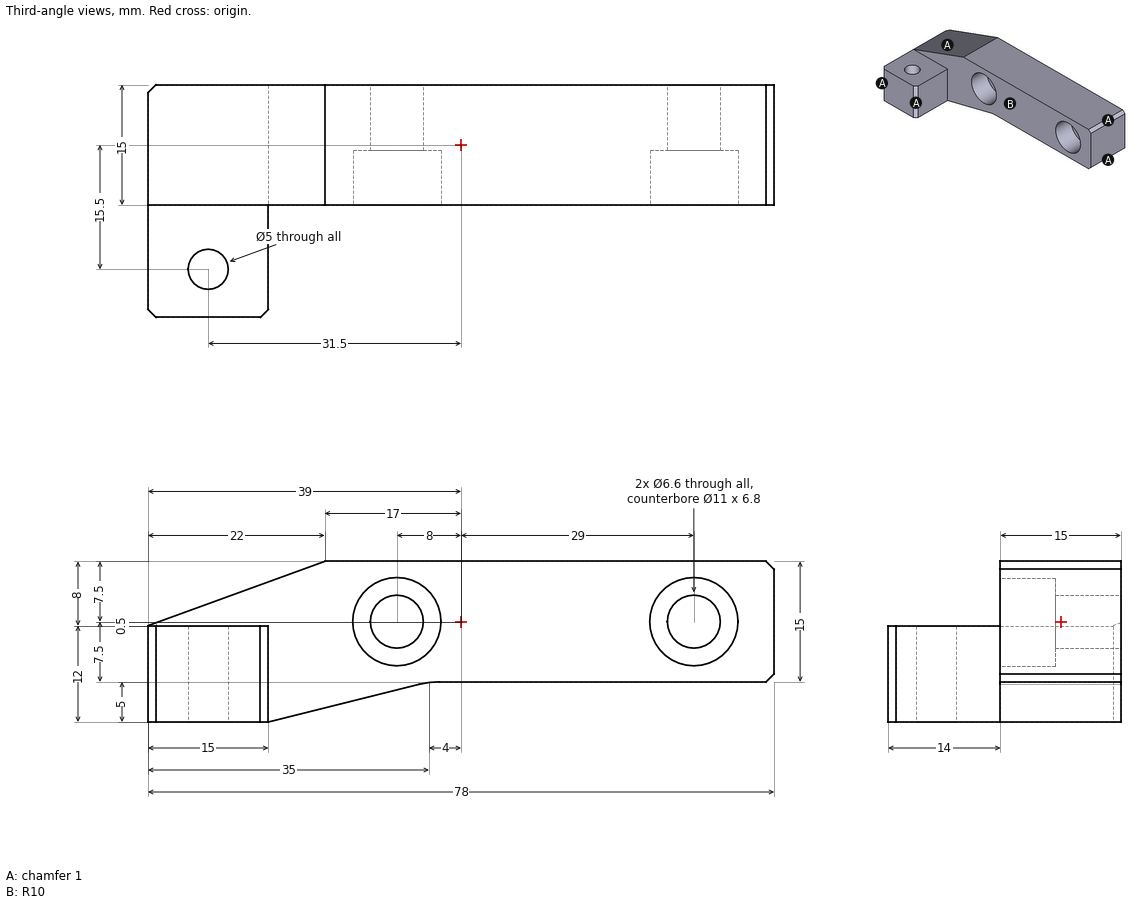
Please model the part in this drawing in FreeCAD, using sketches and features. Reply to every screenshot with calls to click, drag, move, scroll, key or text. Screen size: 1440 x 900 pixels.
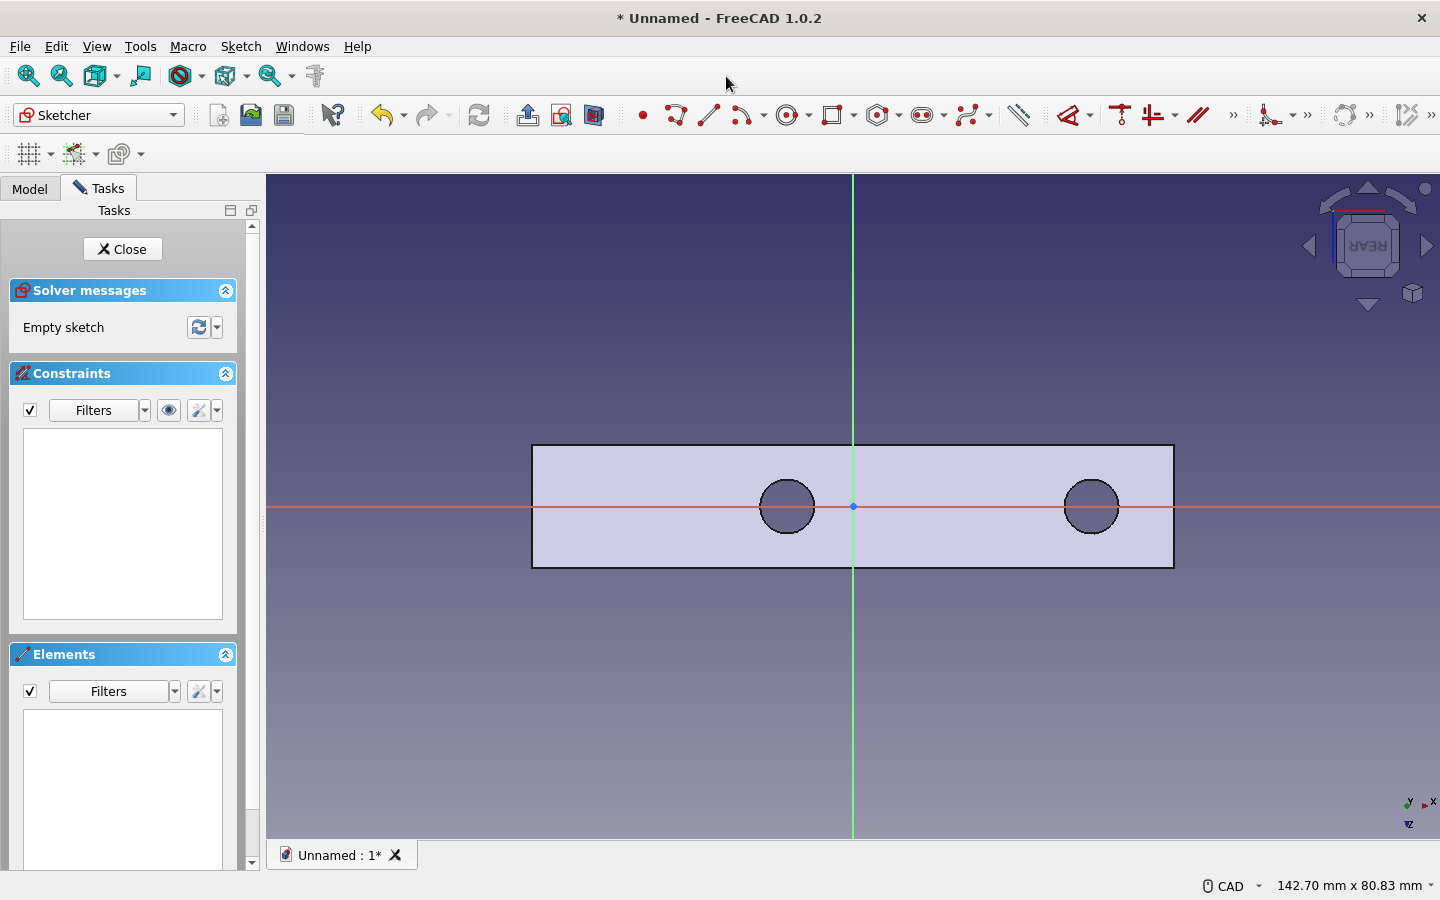
scroll(618, 413, up, 4)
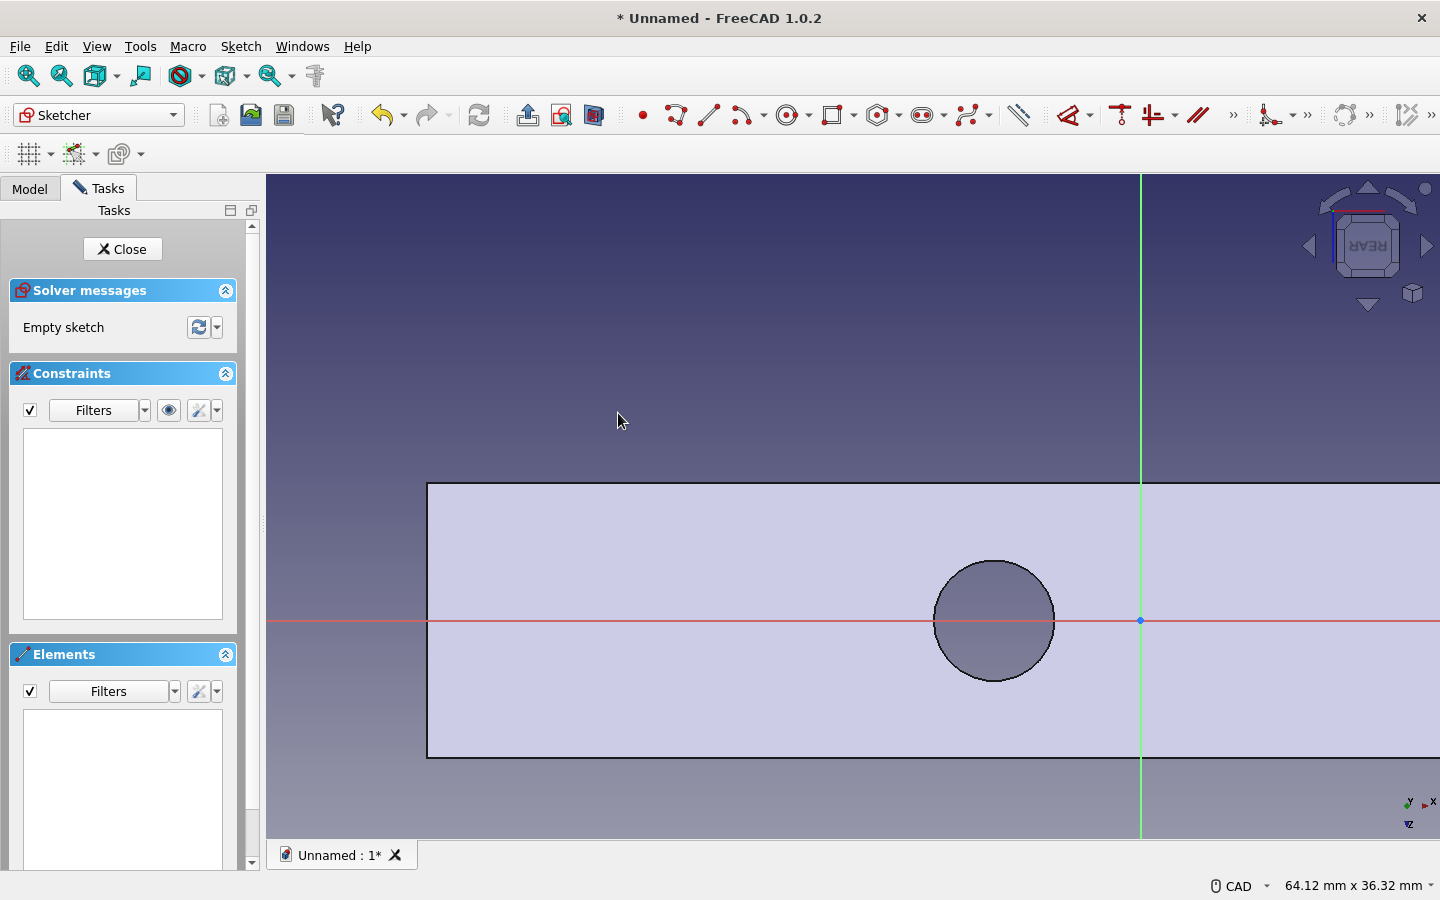
key(g)
key(m)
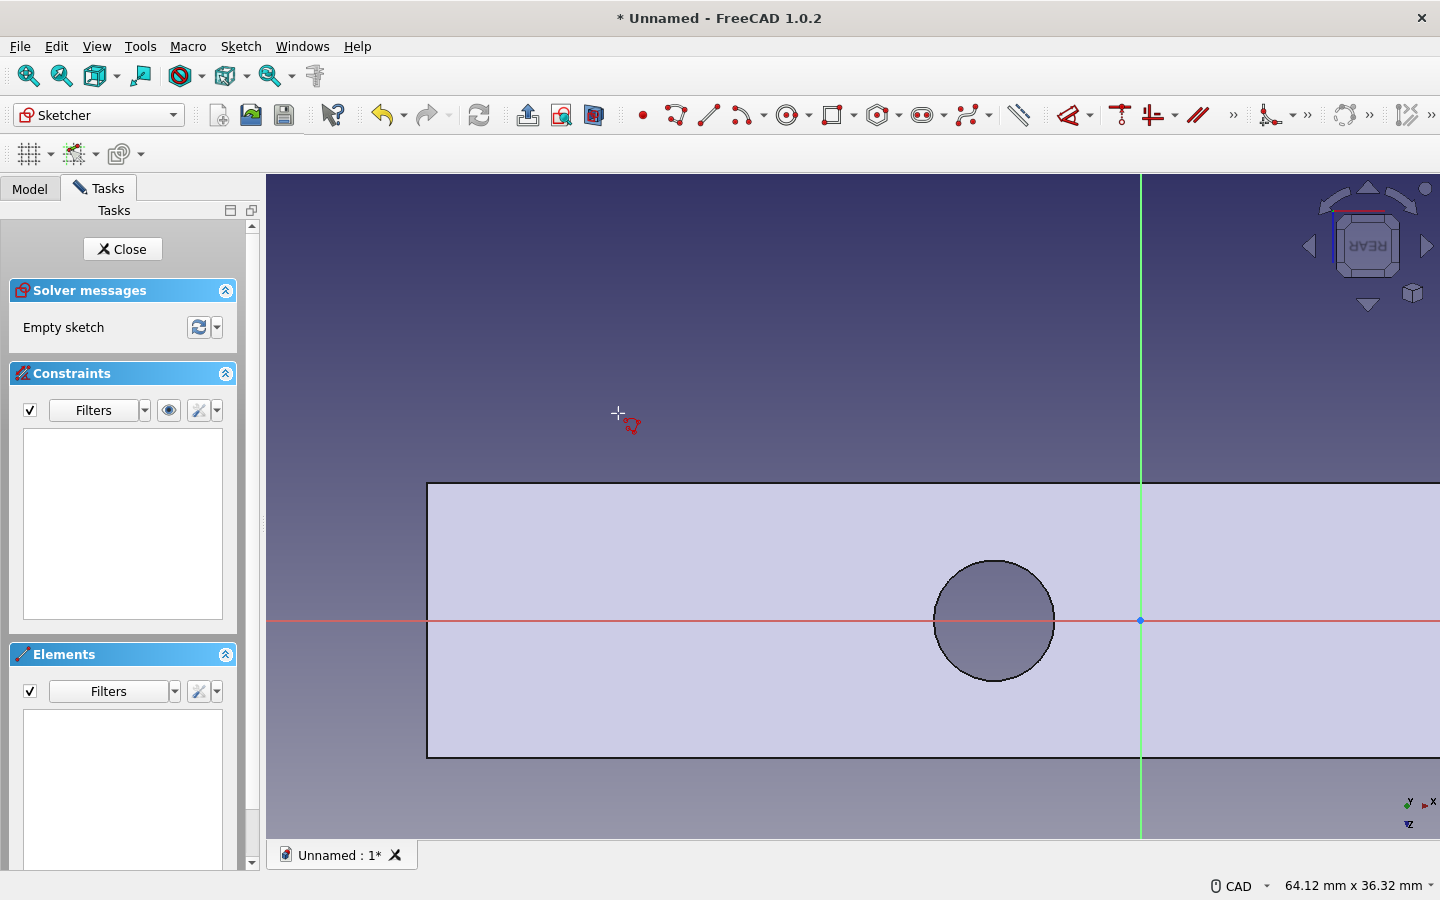
click(1067, 483)
click(701, 392)
click(427, 392)
click(427, 483)
click(1067, 484)
key(Escape)
key(Escape)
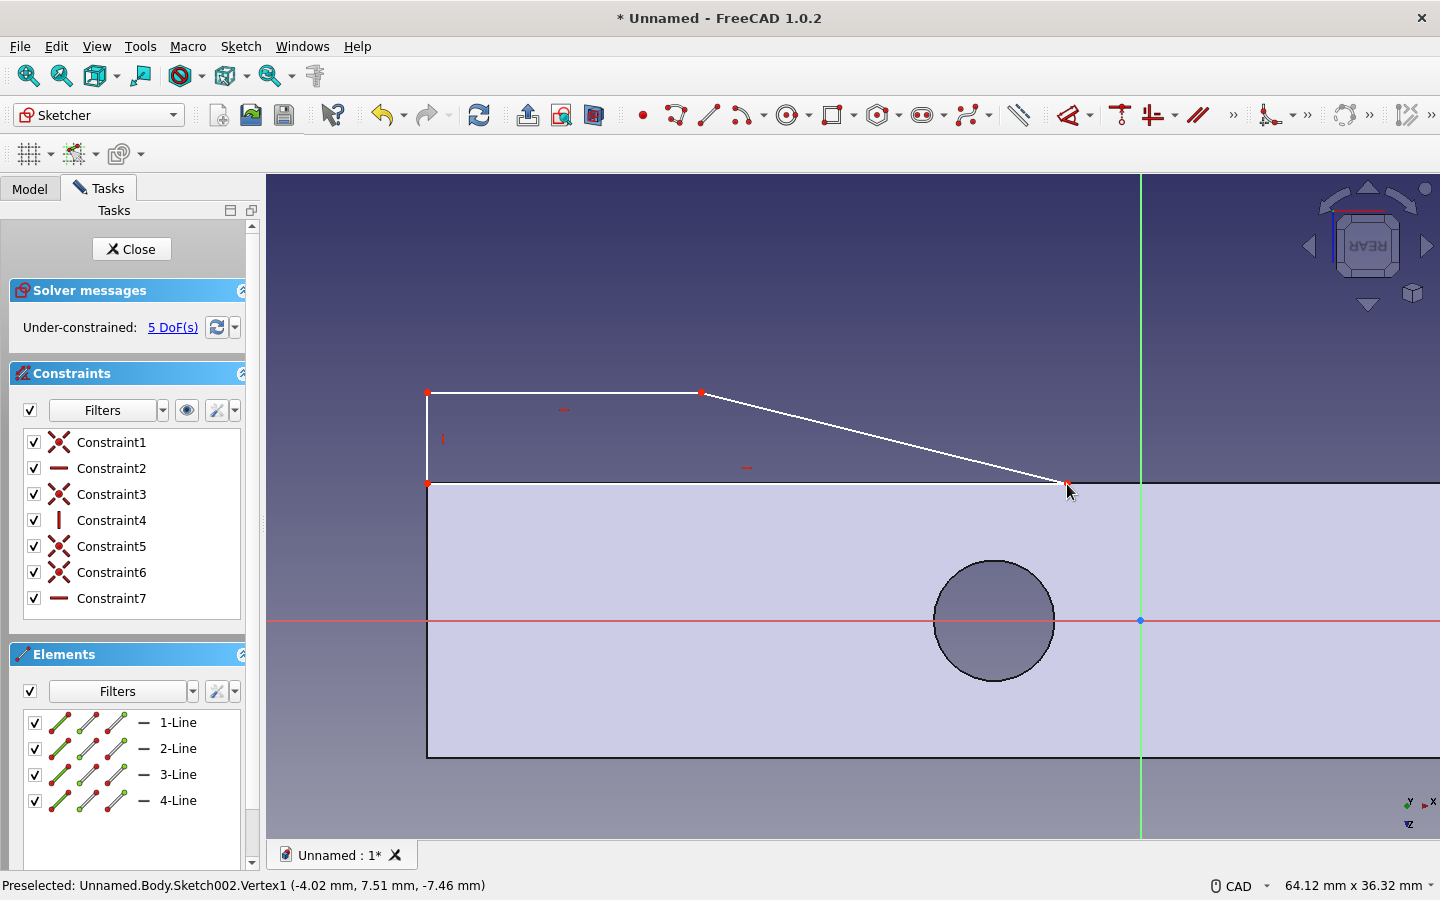
click(427, 420)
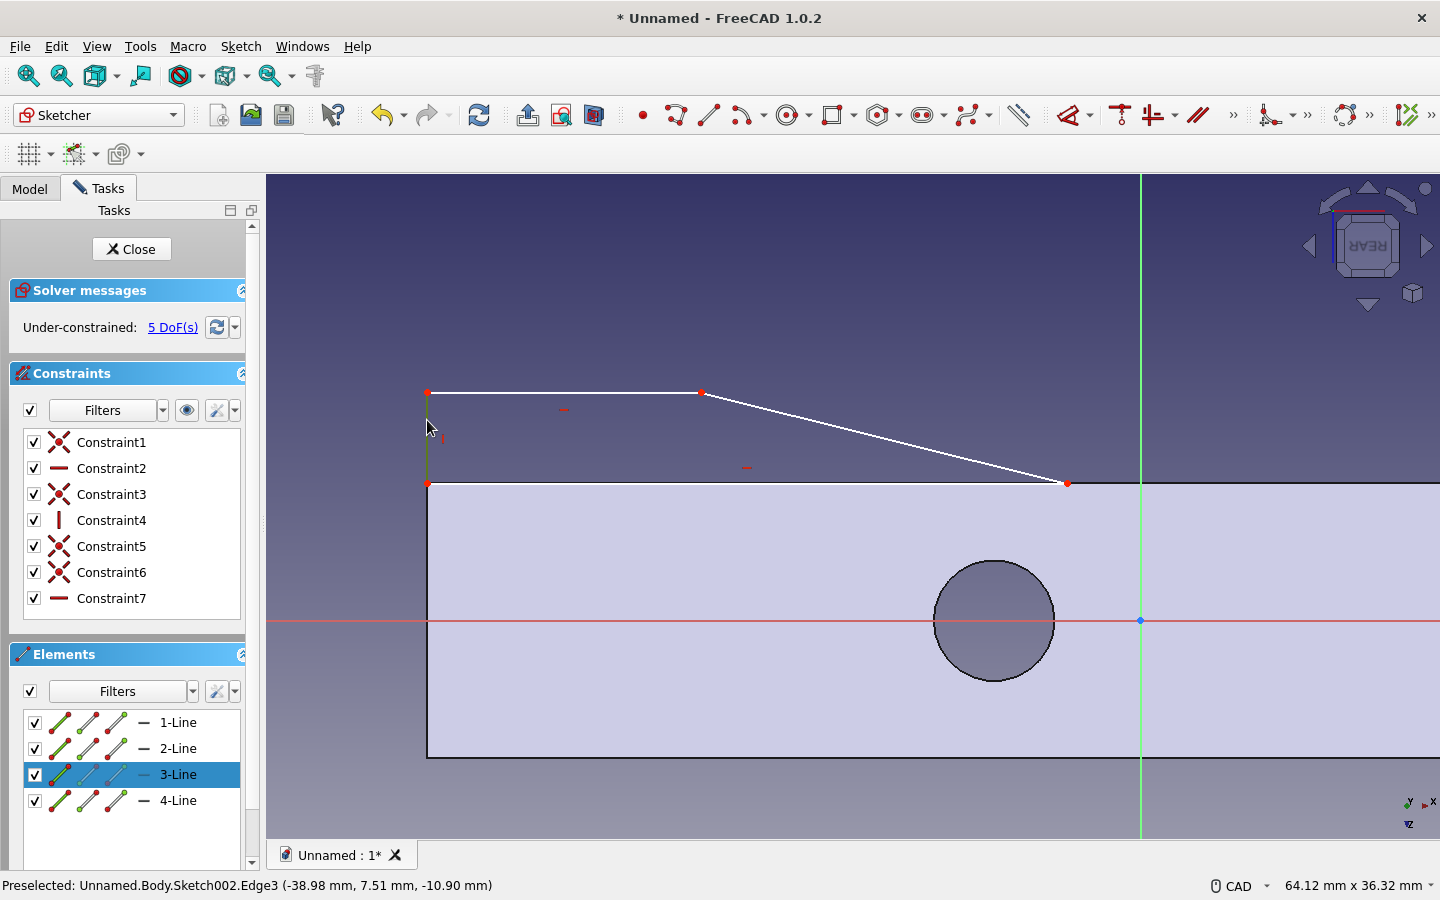
key(i)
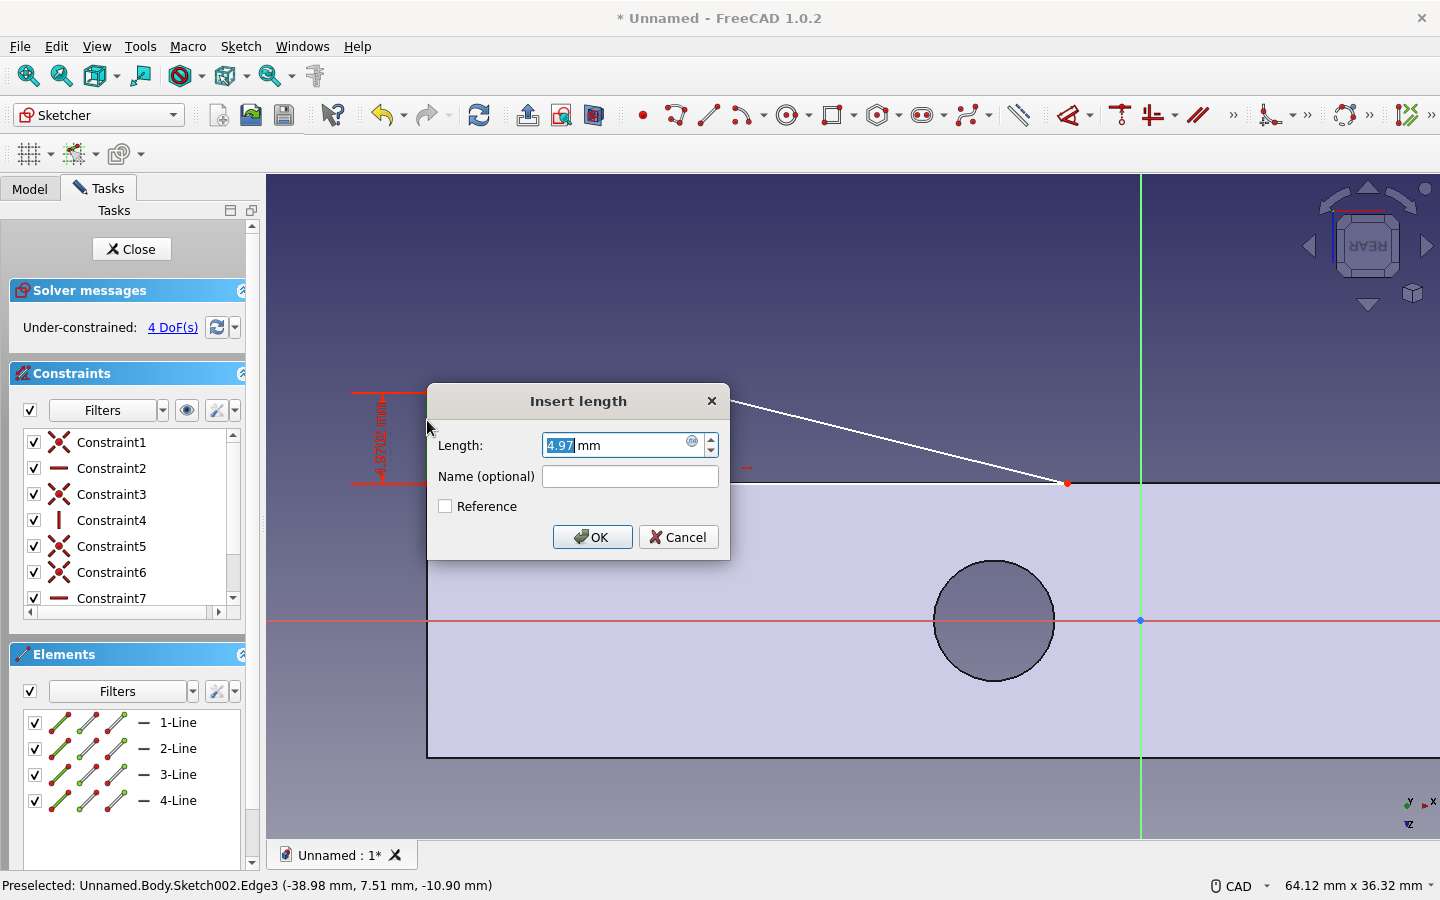
text(5)
key(Return)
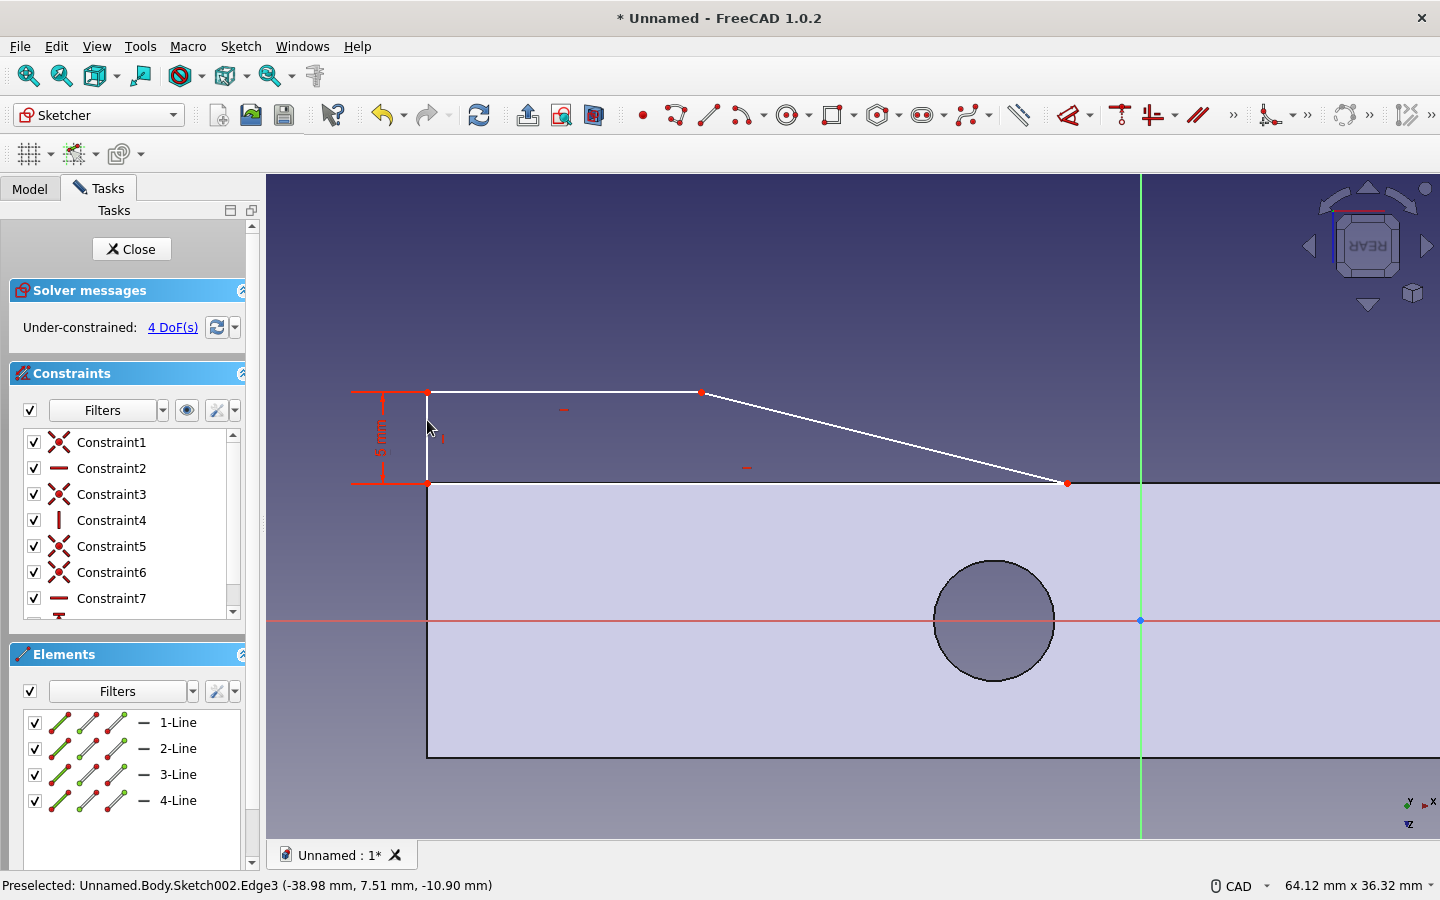
click(619, 392)